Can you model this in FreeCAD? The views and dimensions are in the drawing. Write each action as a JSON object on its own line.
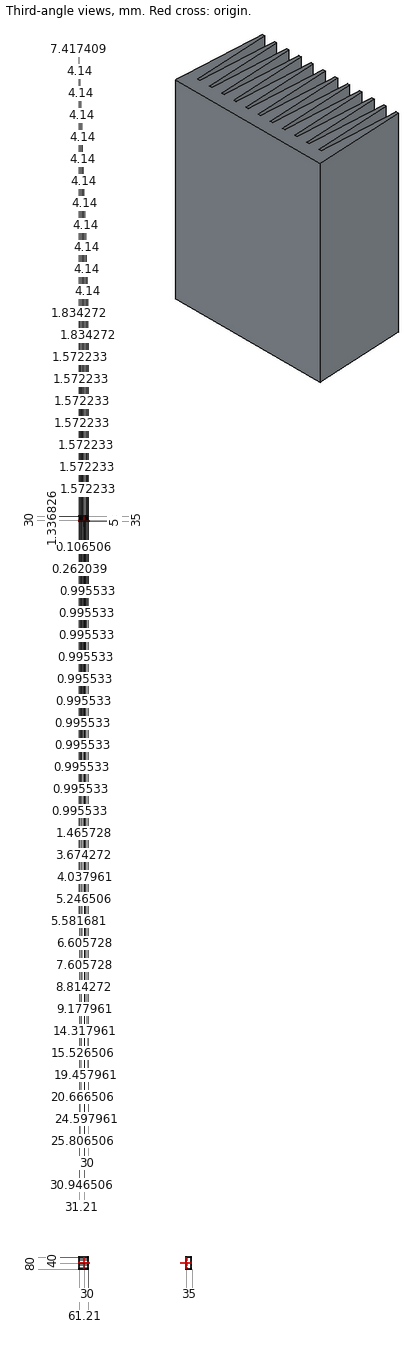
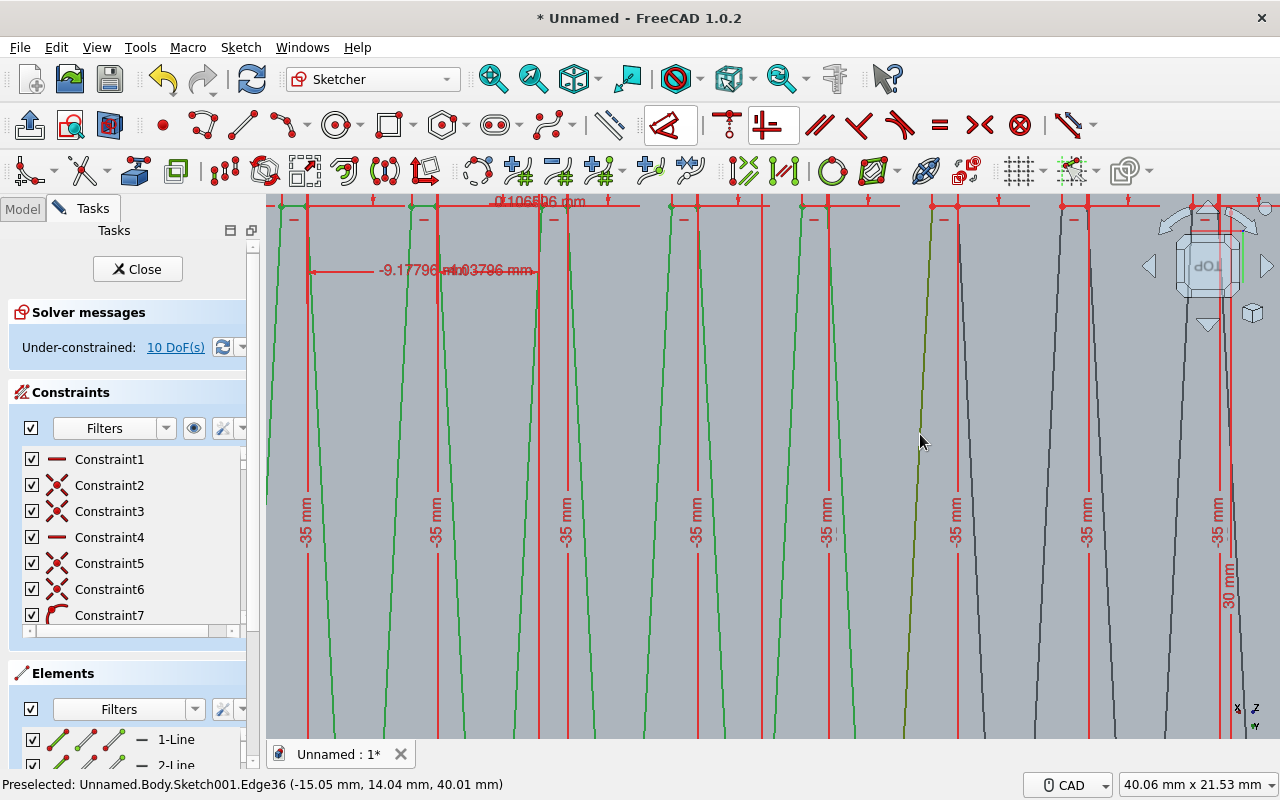
{"action": "key", "text": "l"}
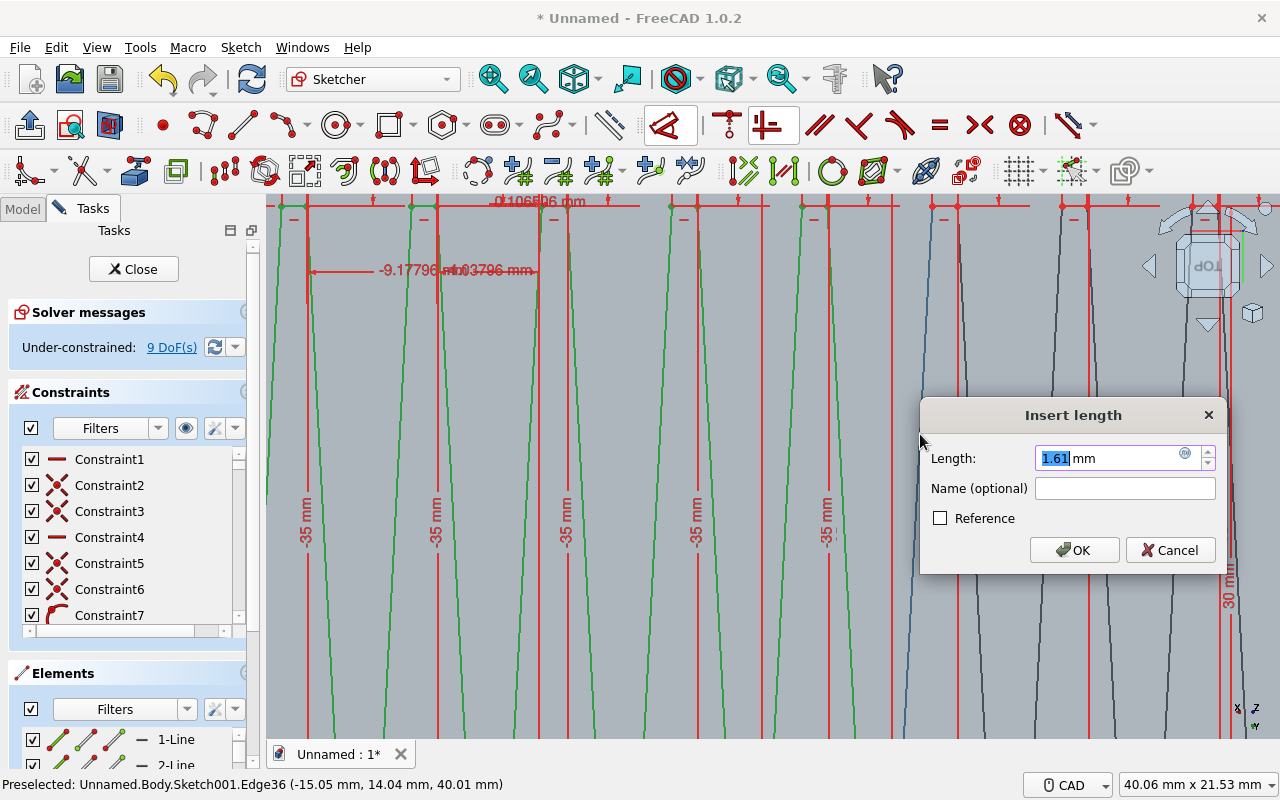
{"action": "type", "text": "1.572233"}
{"action": "key", "text": "Return"}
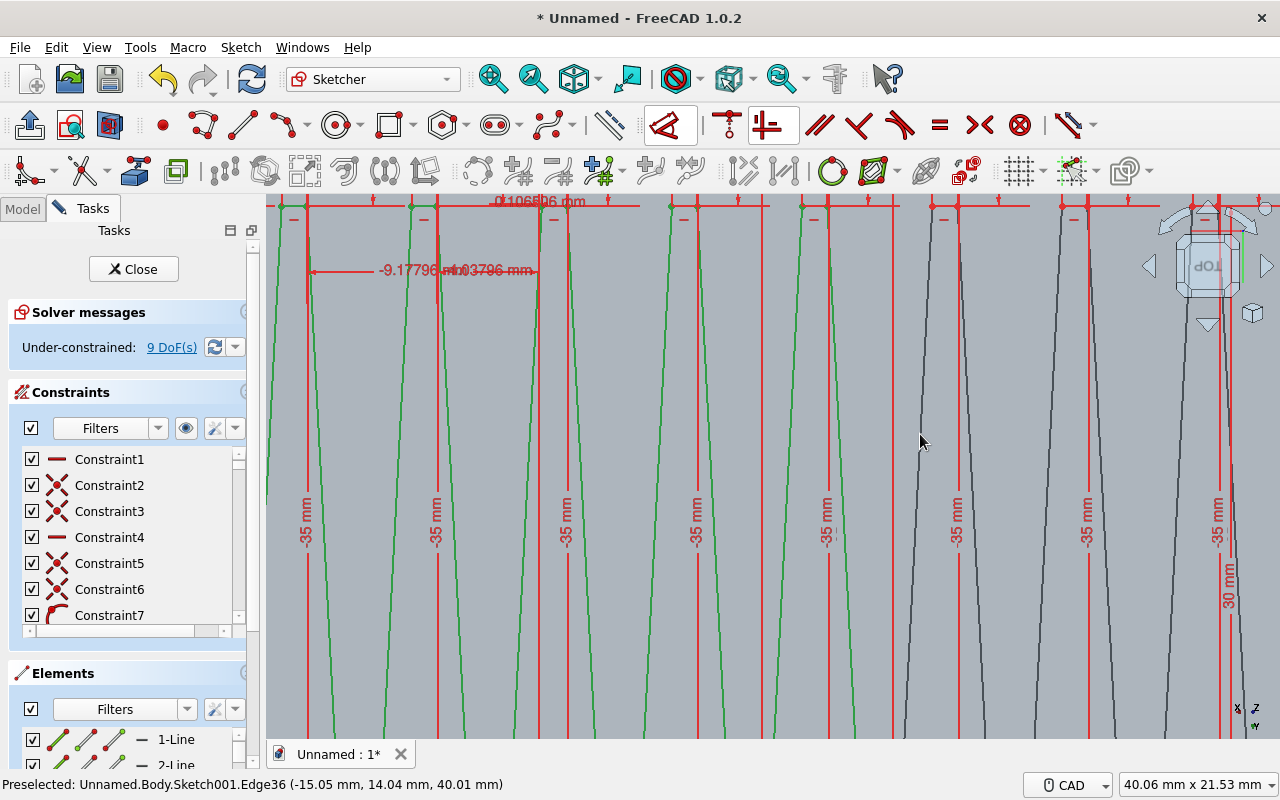
{"action": "left_click", "coordinate": [1050, 434]}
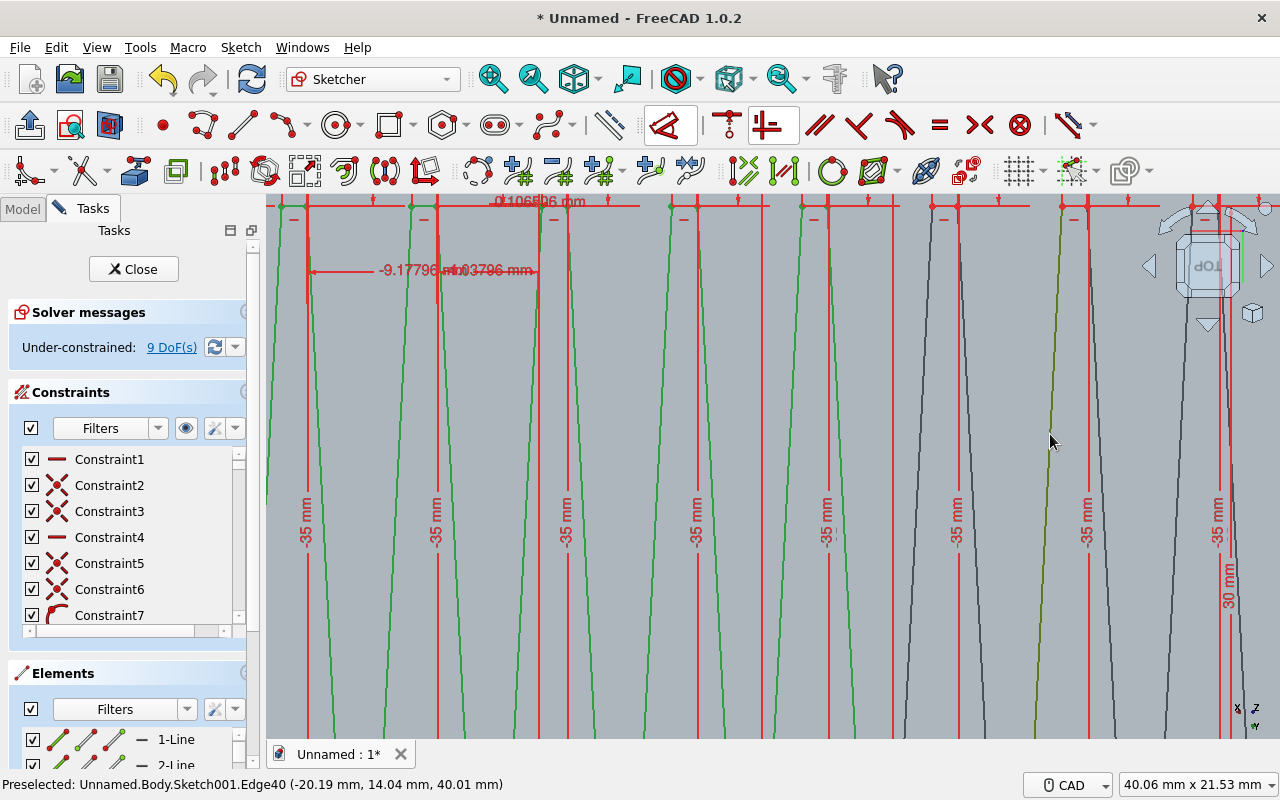
{"action": "left_click", "coordinate": [692, 126]}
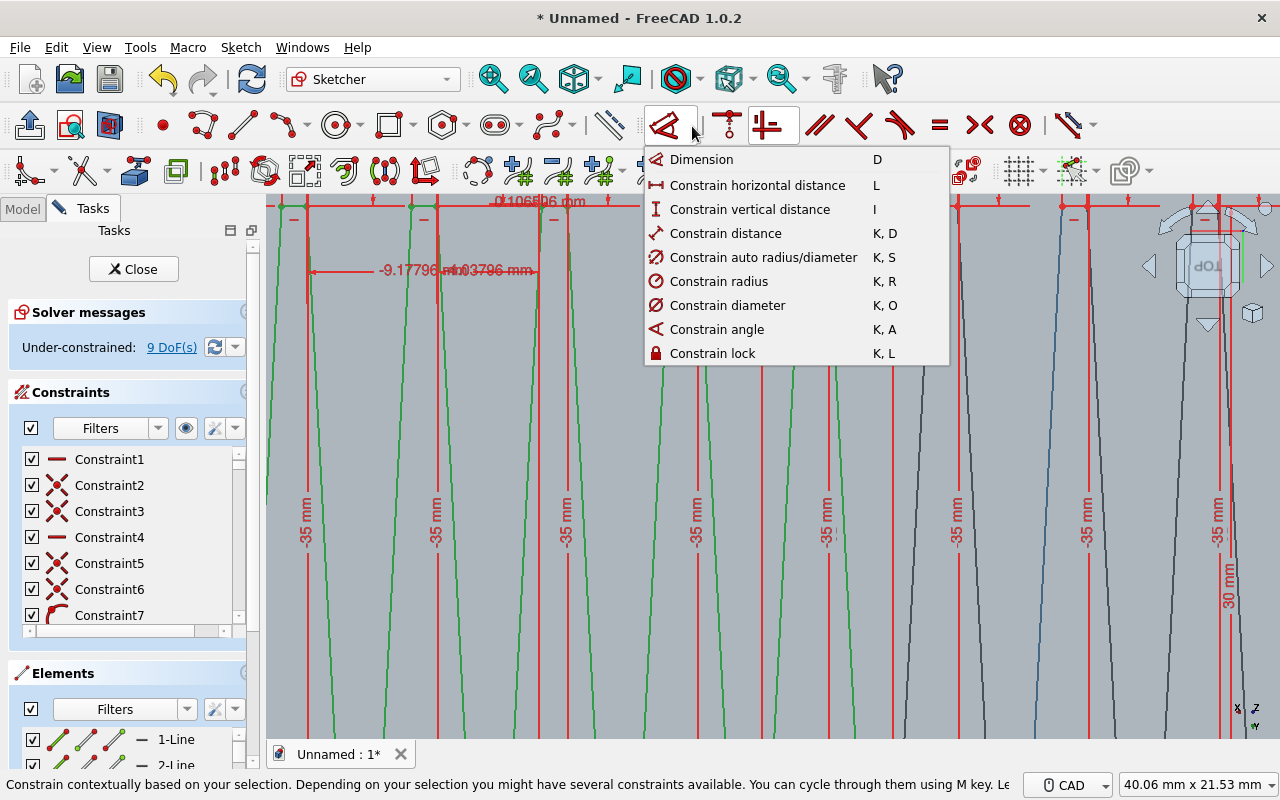
{"action": "left_click", "coordinate": [797, 185]}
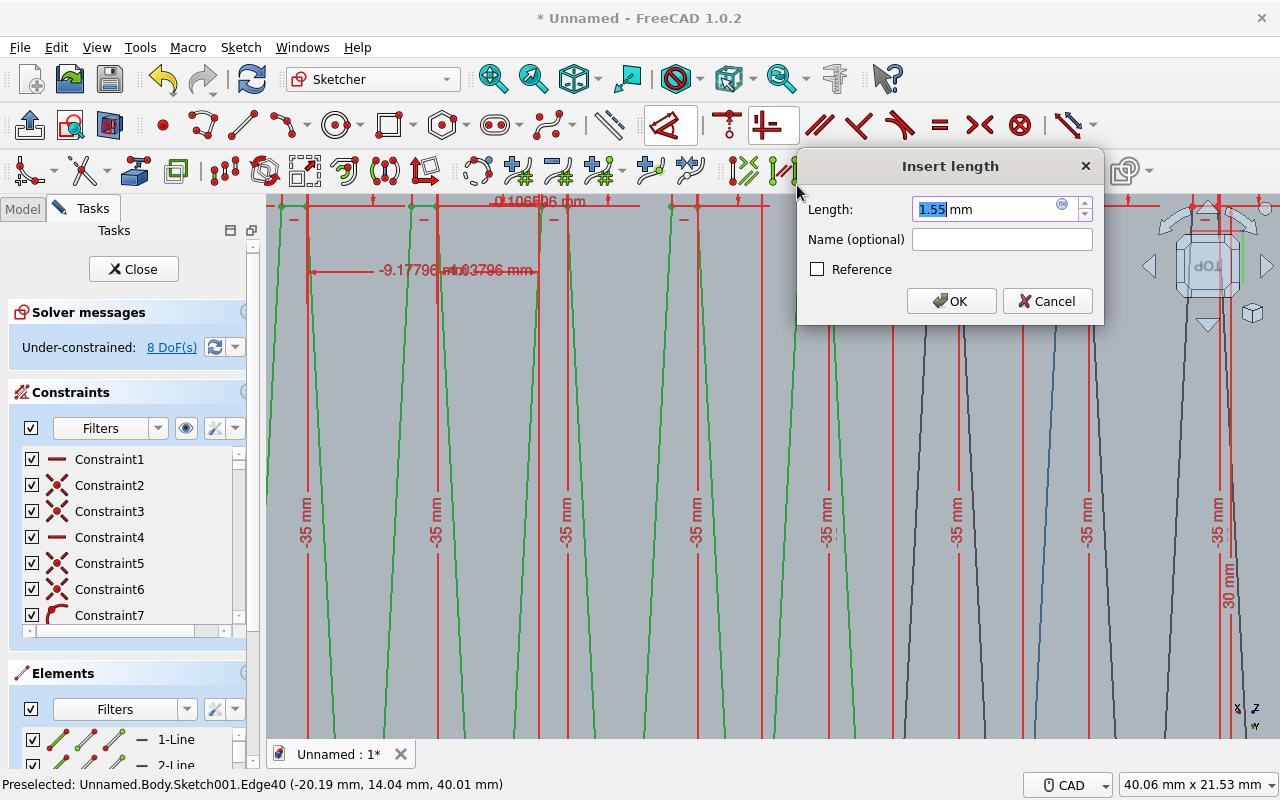
{"action": "type", "text": "1.572233"}
{"action": "key", "text": "Return"}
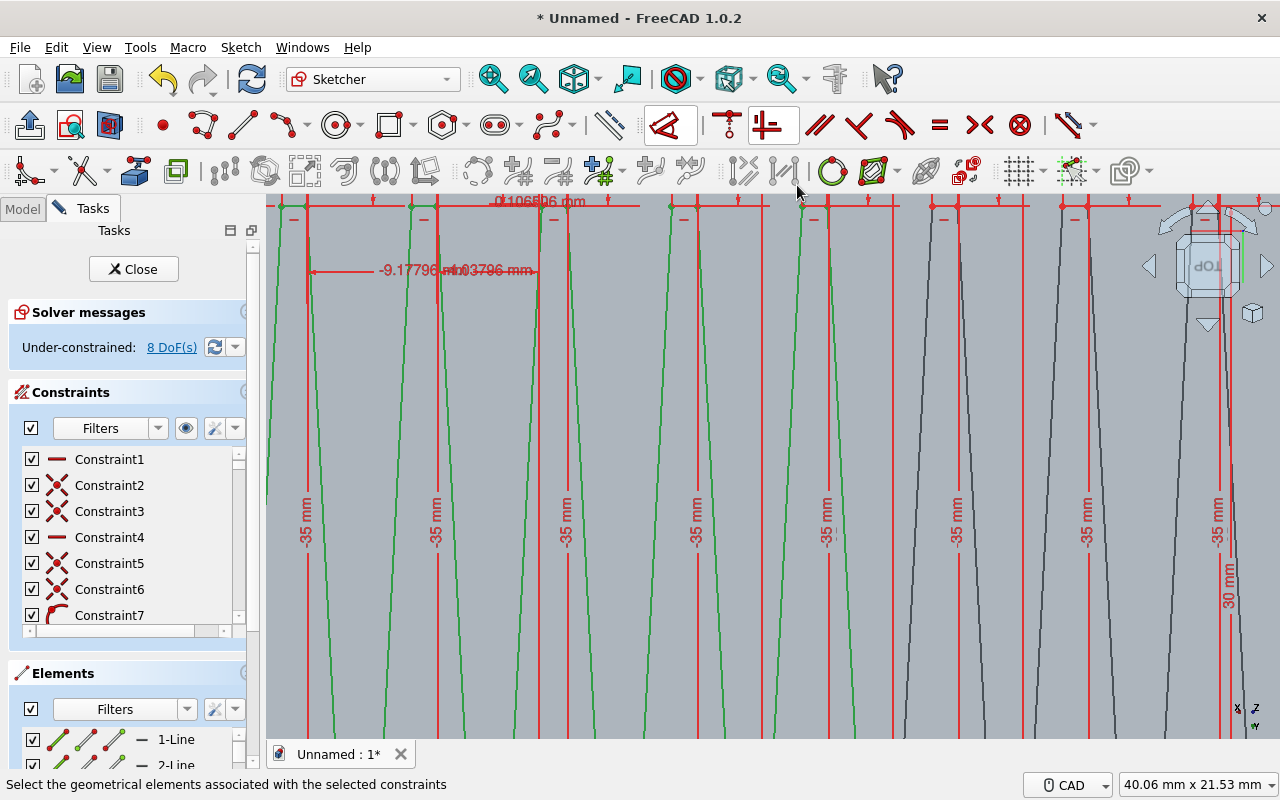
{"action": "scroll", "coordinate": [792, 434], "scroll_direction": "down", "scroll_amount": 5}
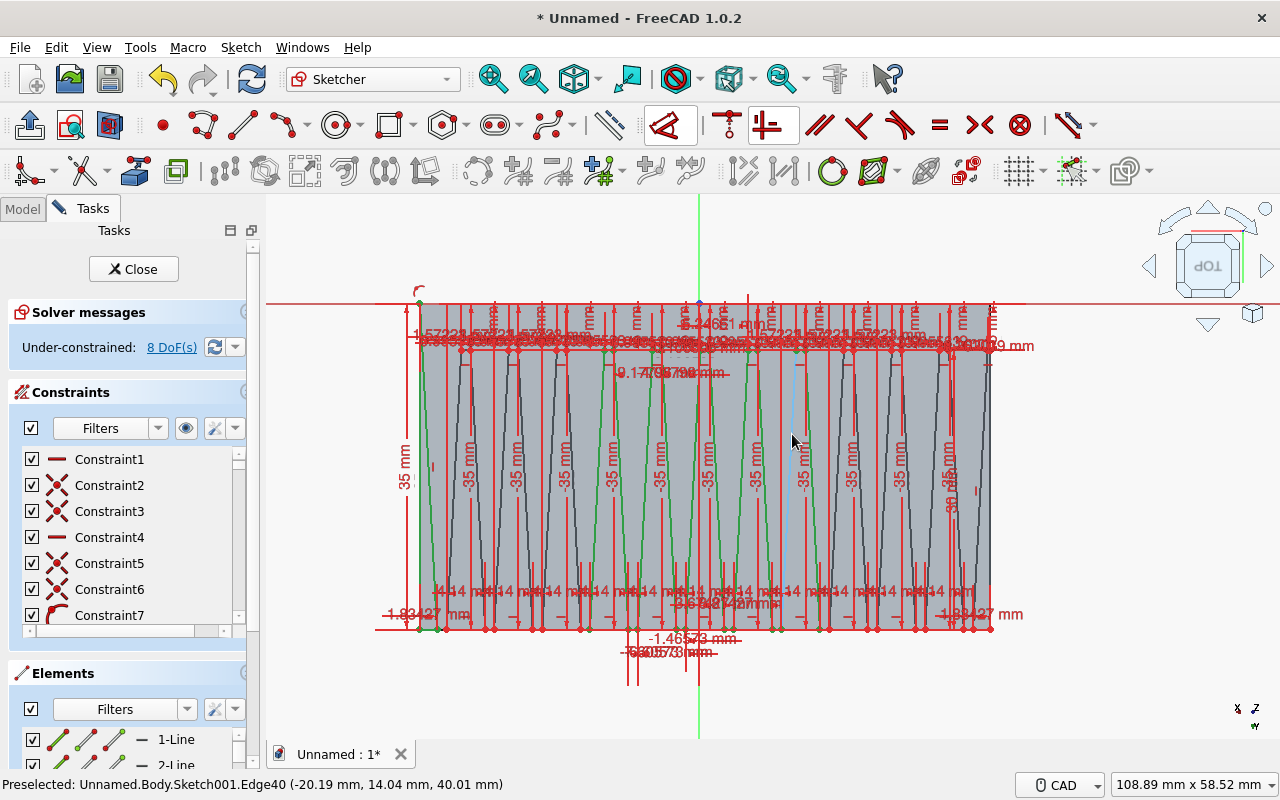
{"action": "scroll", "coordinate": [935, 434], "scroll_direction": "up", "scroll_amount": 5}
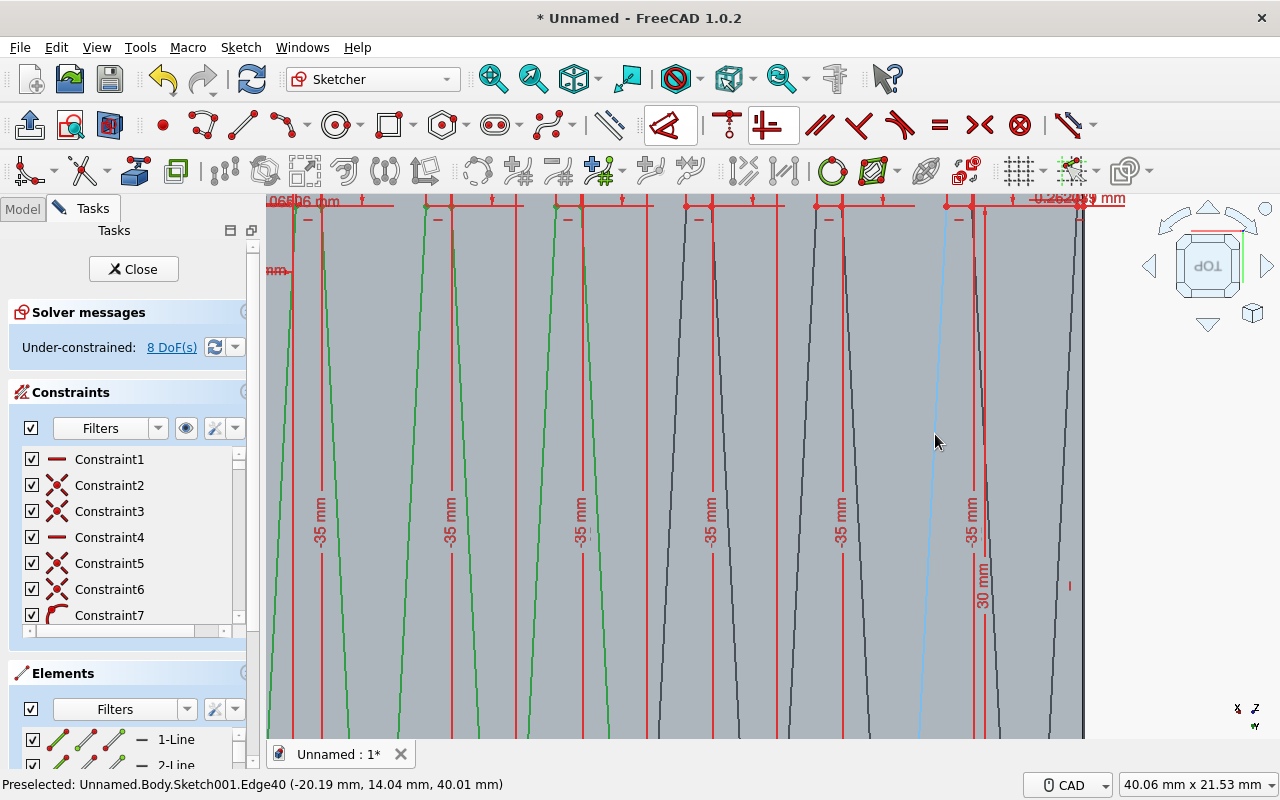
{"action": "left_click", "coordinate": [935, 434]}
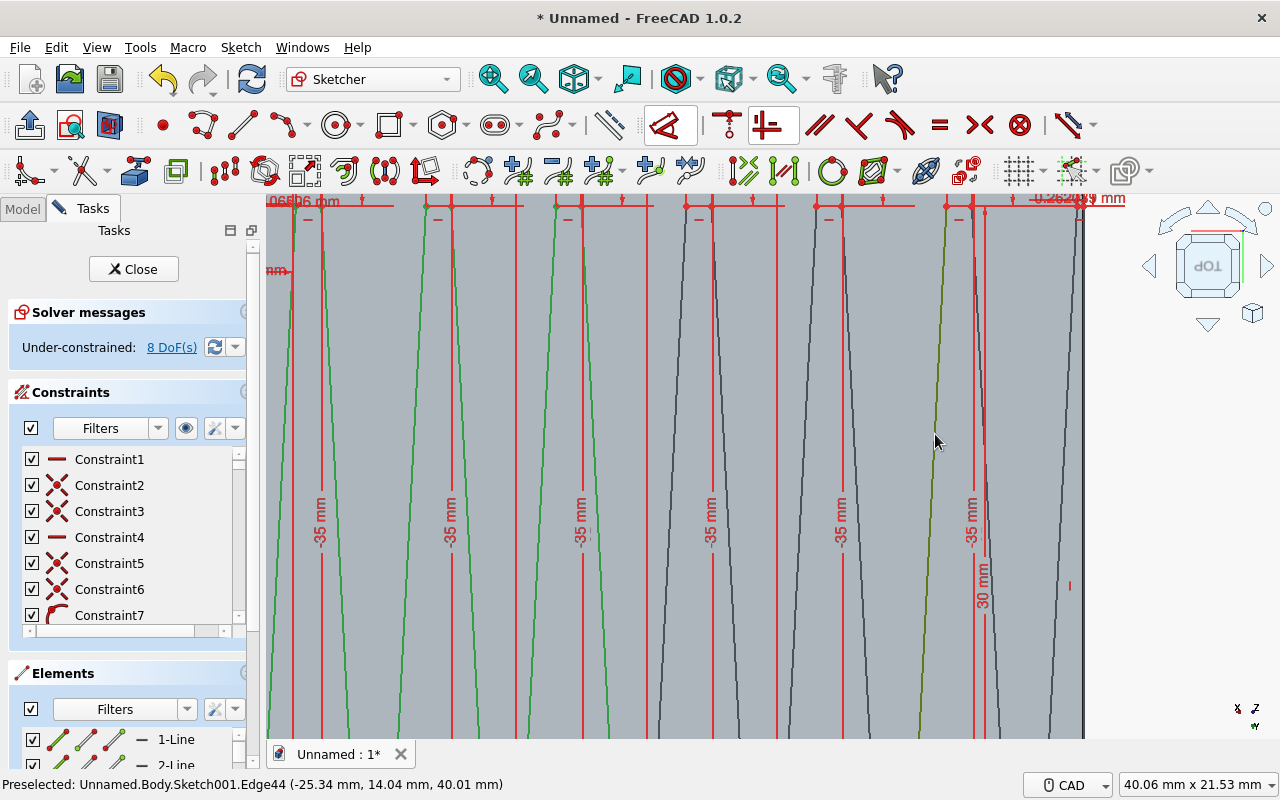
{"action": "left_click", "coordinate": [692, 126]}